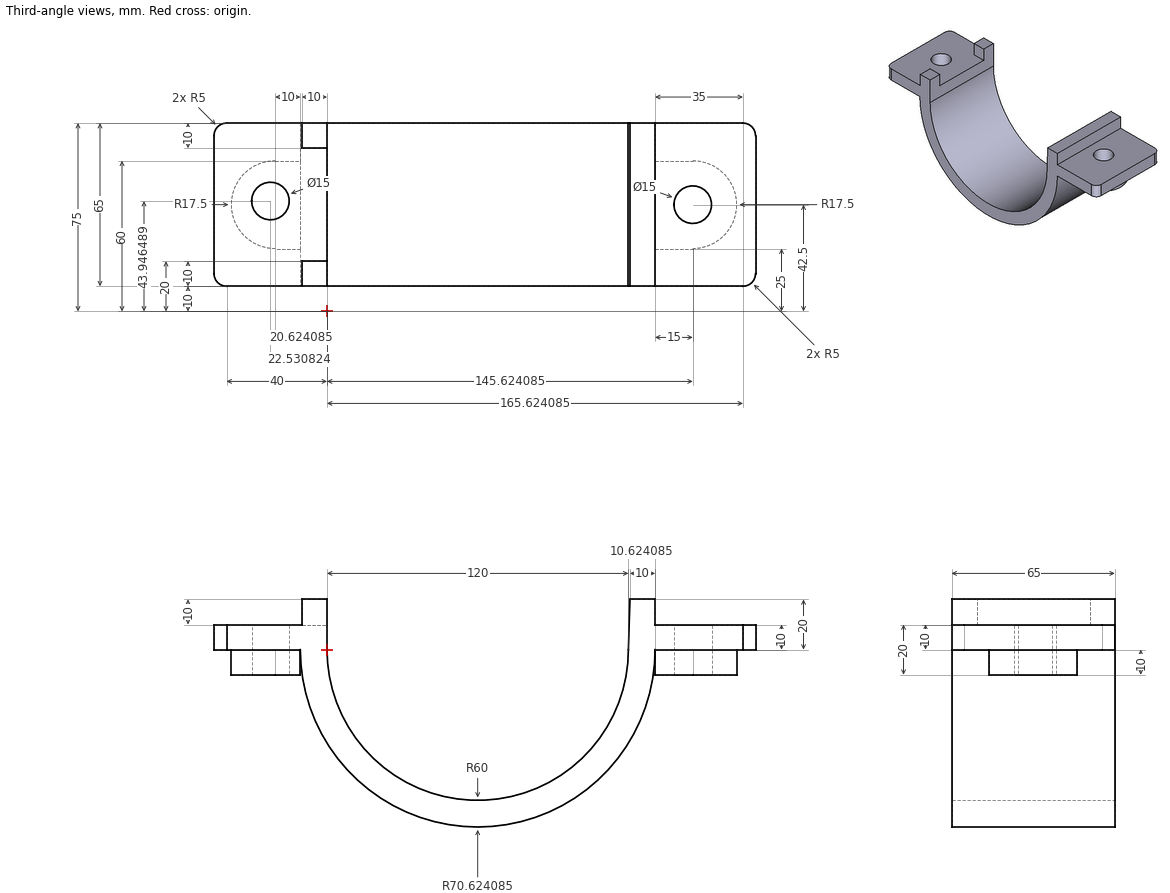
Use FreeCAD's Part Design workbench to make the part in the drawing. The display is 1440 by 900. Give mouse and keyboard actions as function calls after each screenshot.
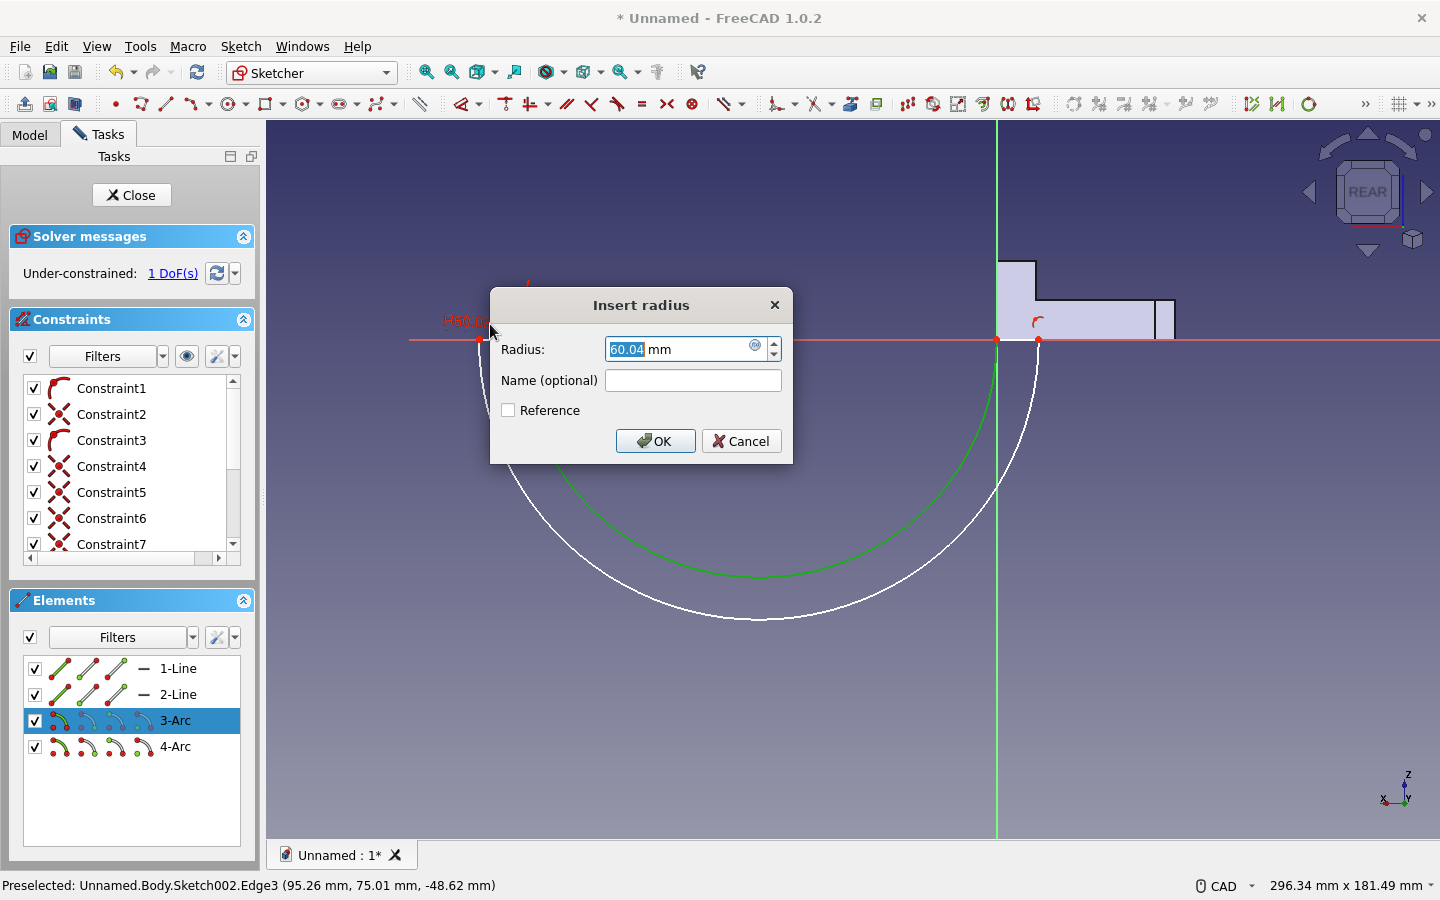
text(60)
key(Return)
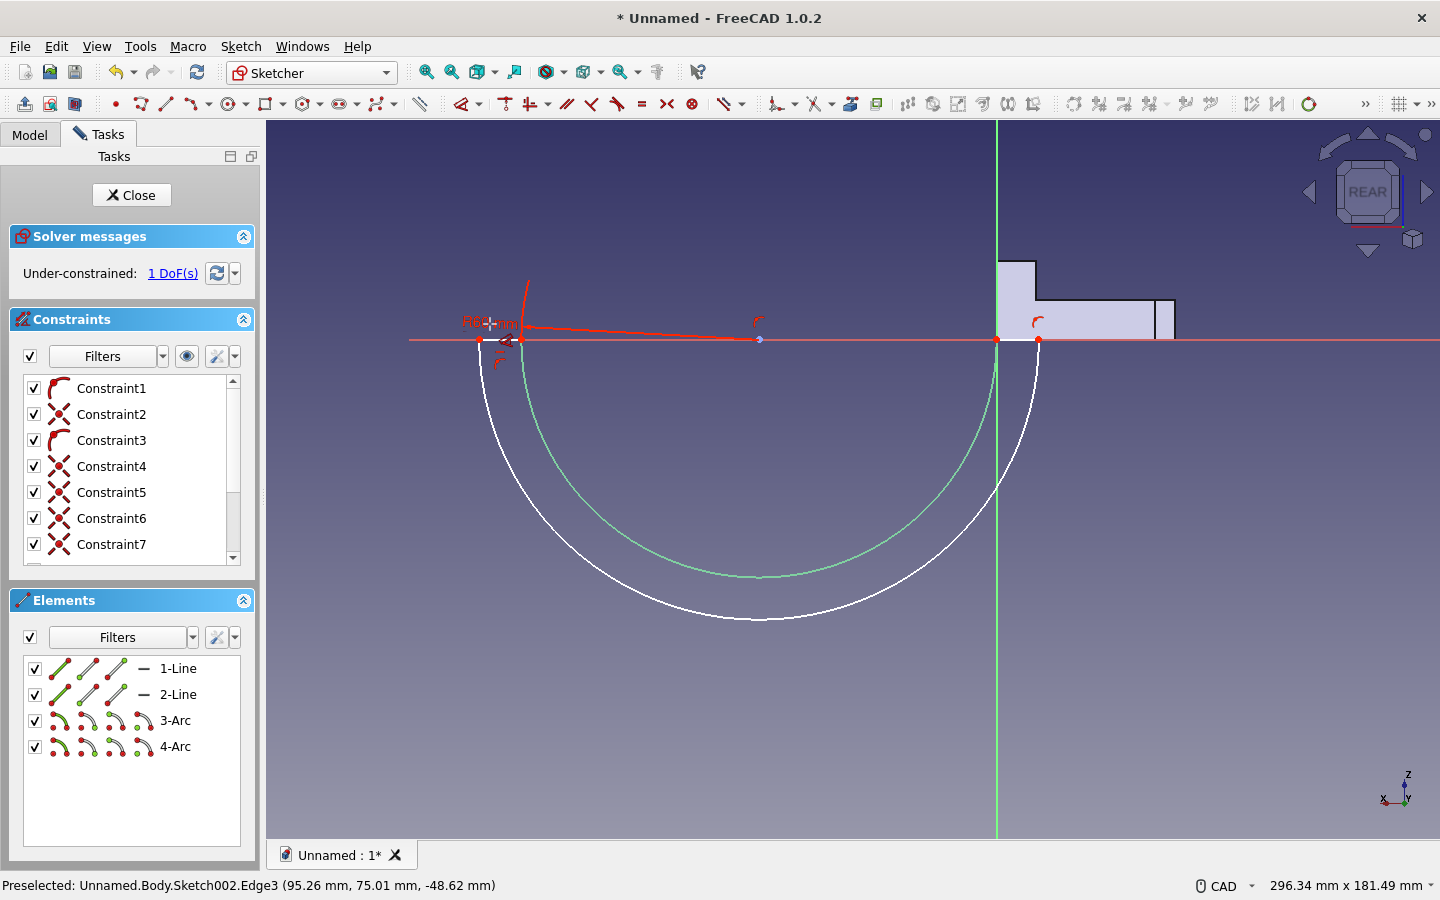
click(595, 566)
click(576, 592)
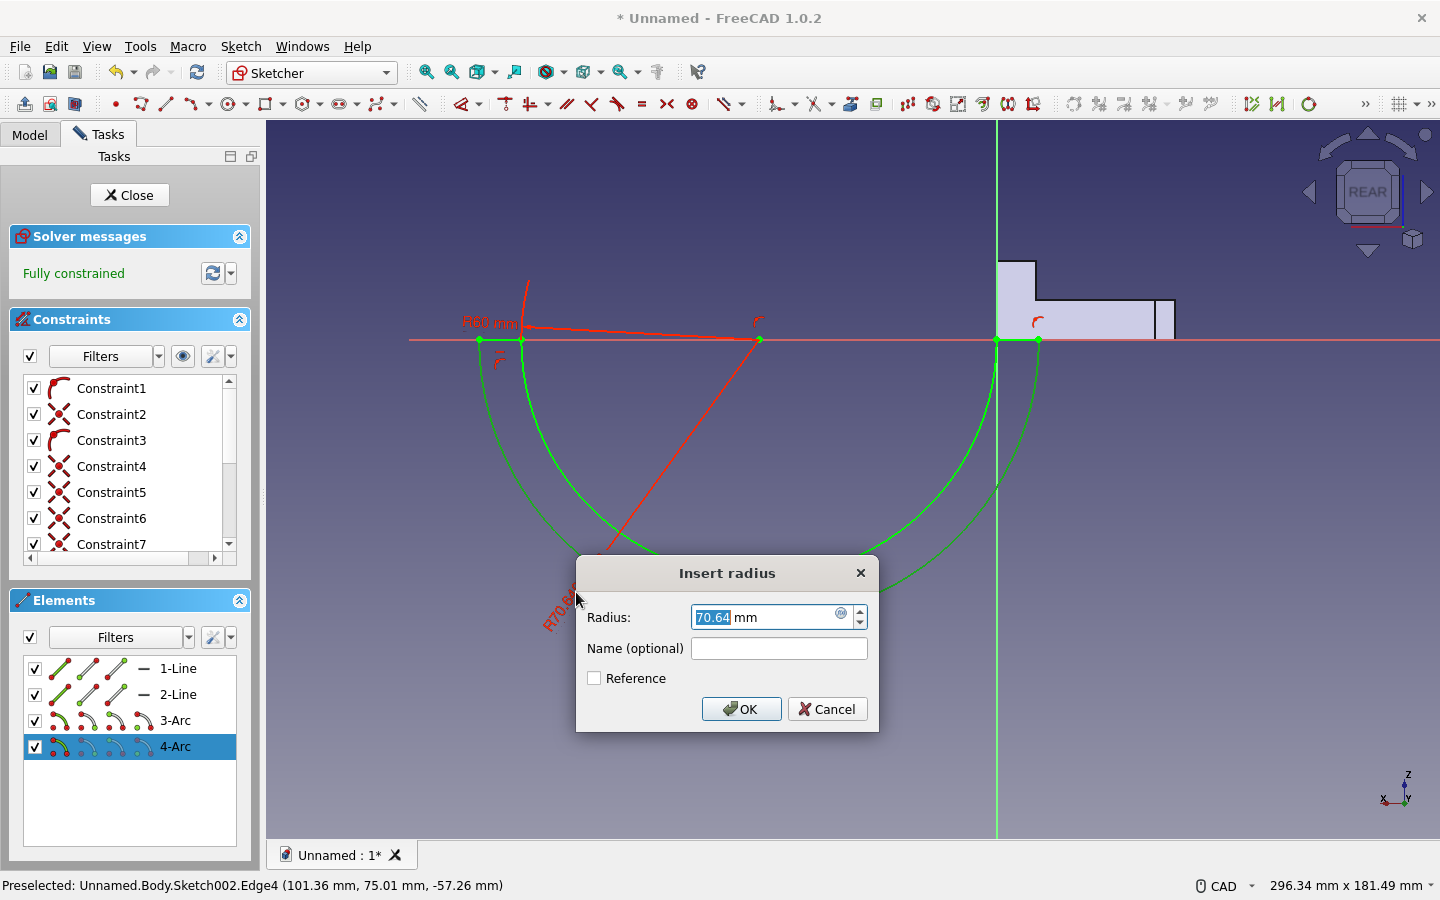
text(70.624085)
key(Return)
key(Escape)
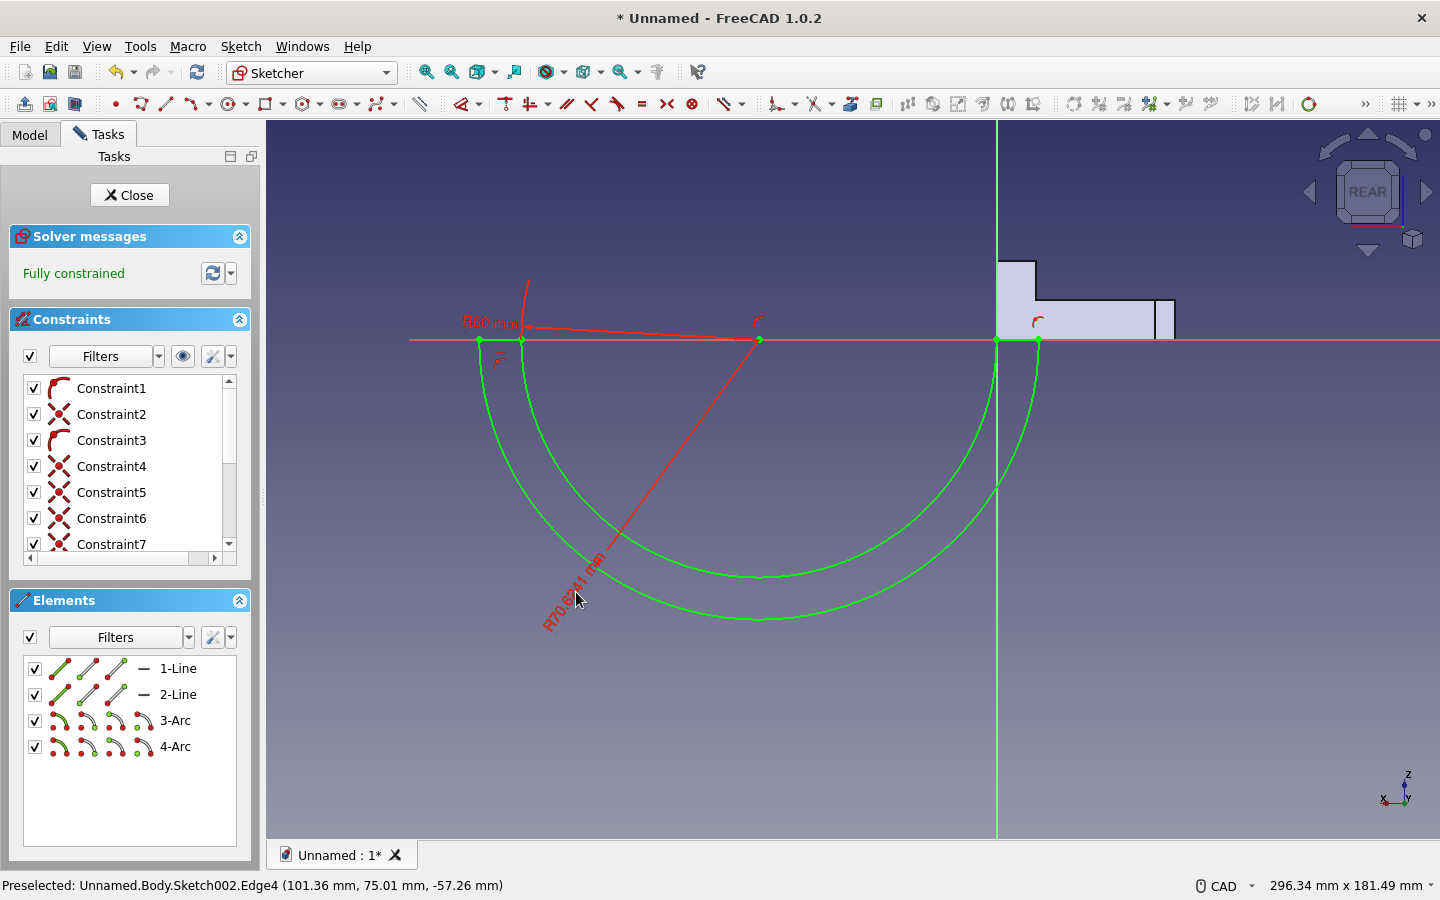
click(130, 195)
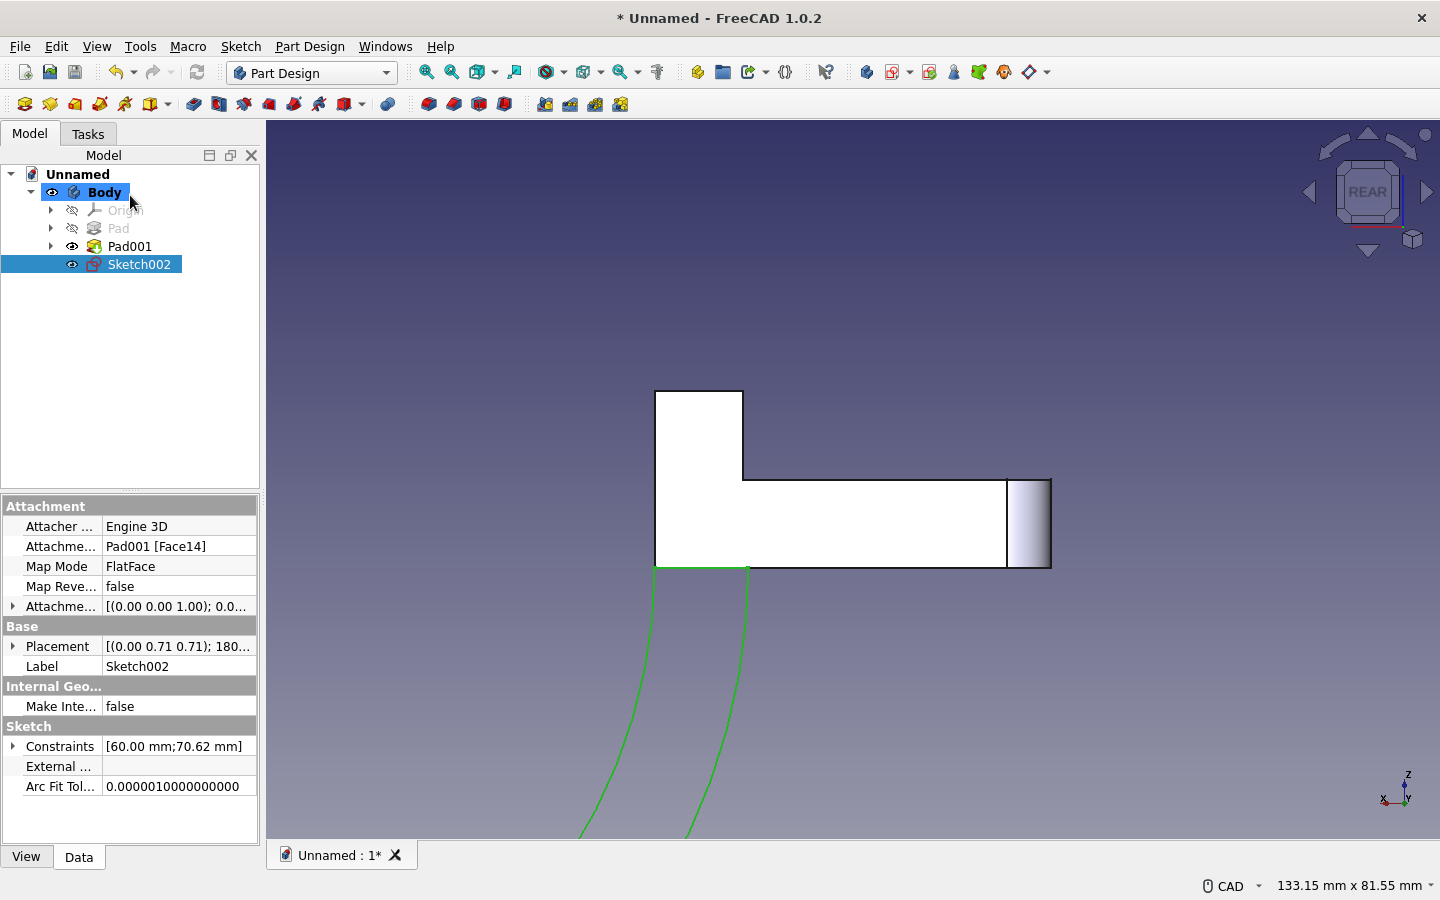
click(25, 104)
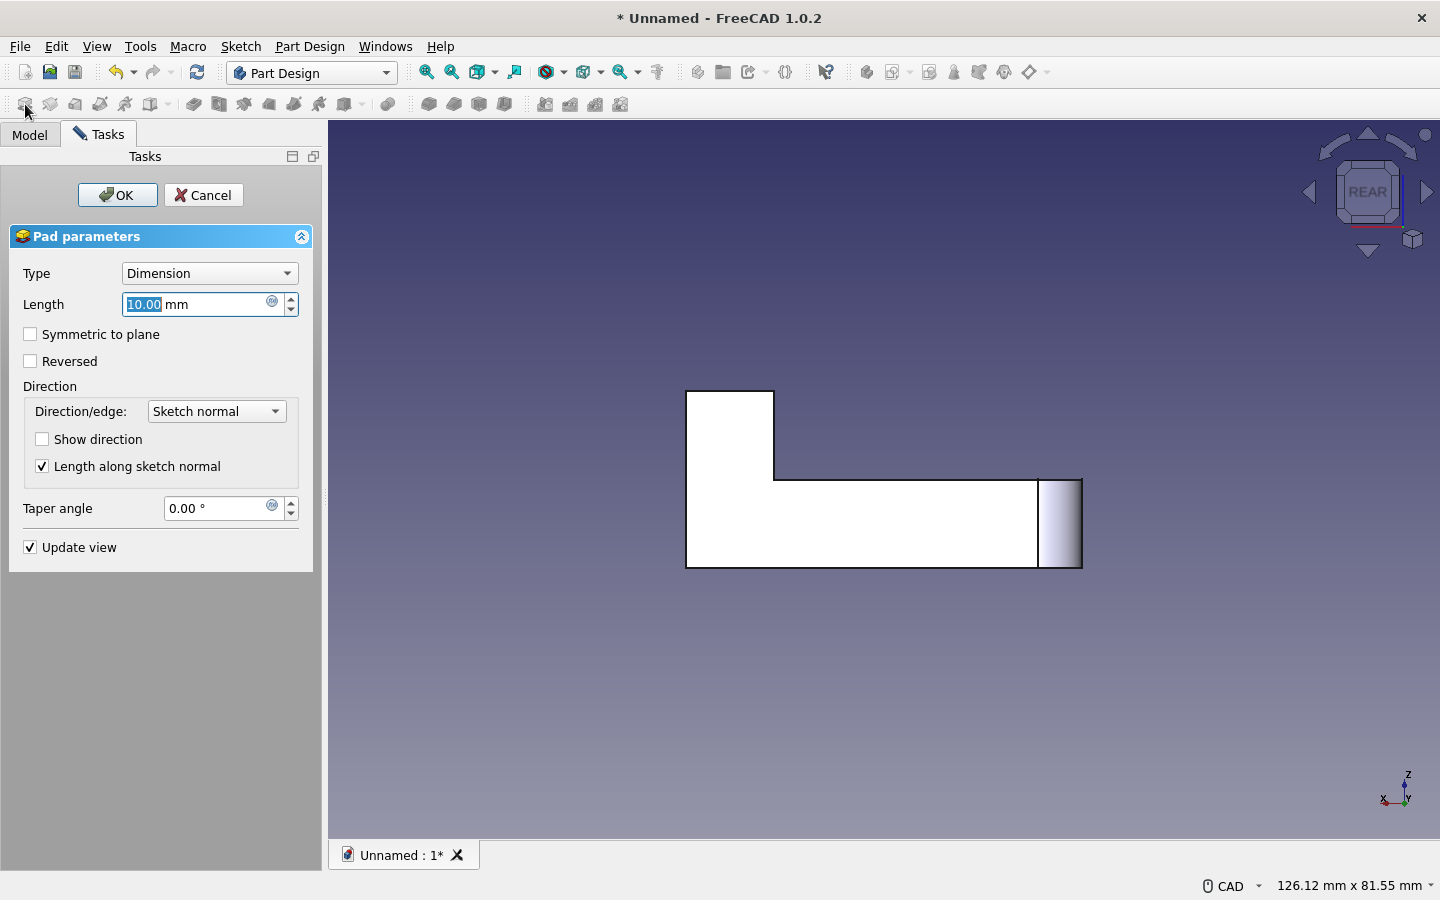
text(65)
key(Tab)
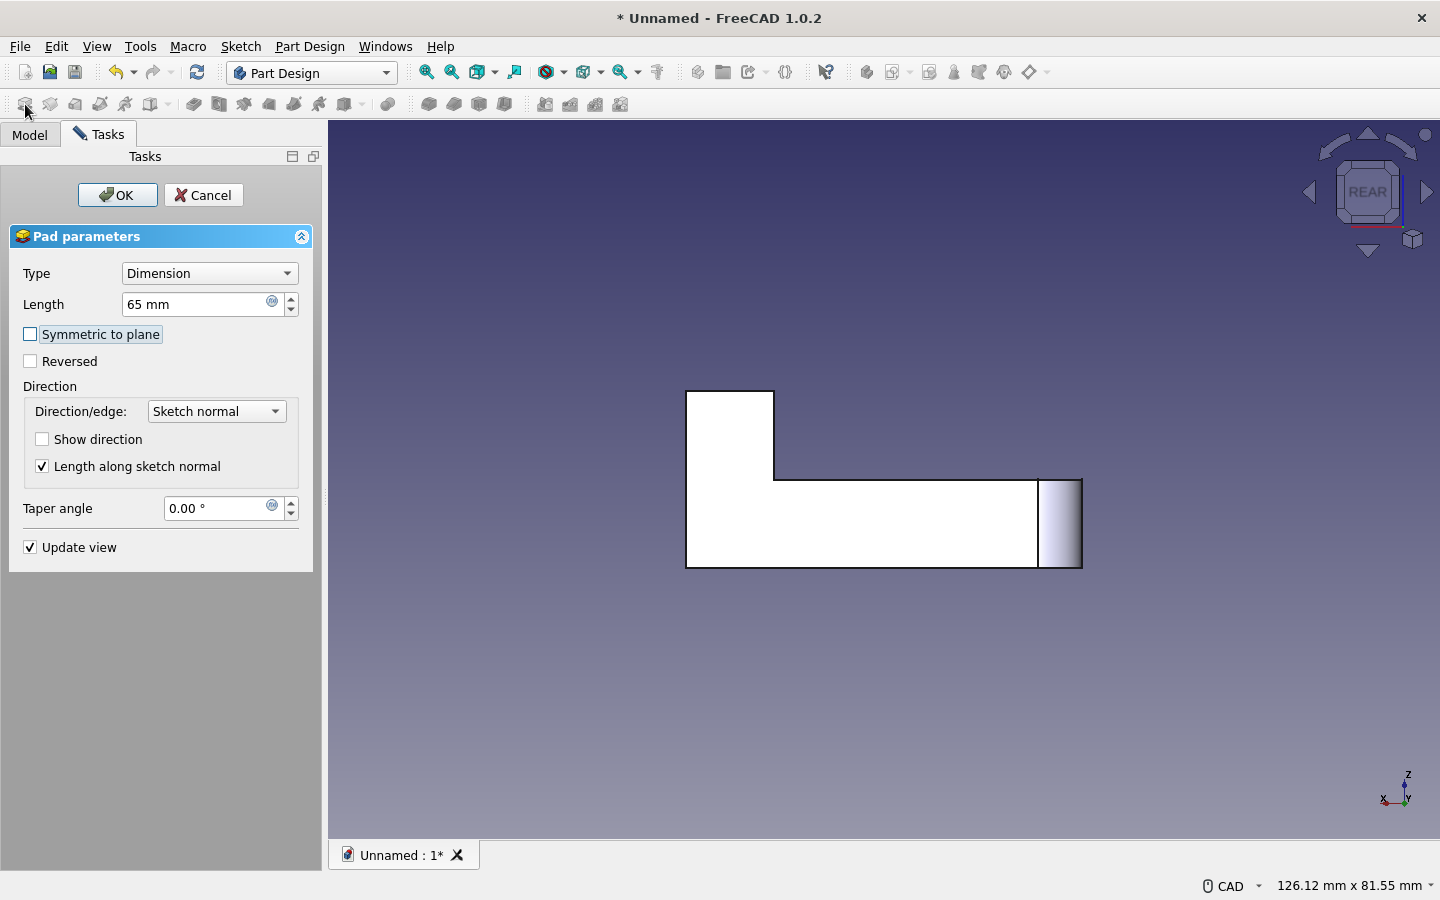
click(31, 361)